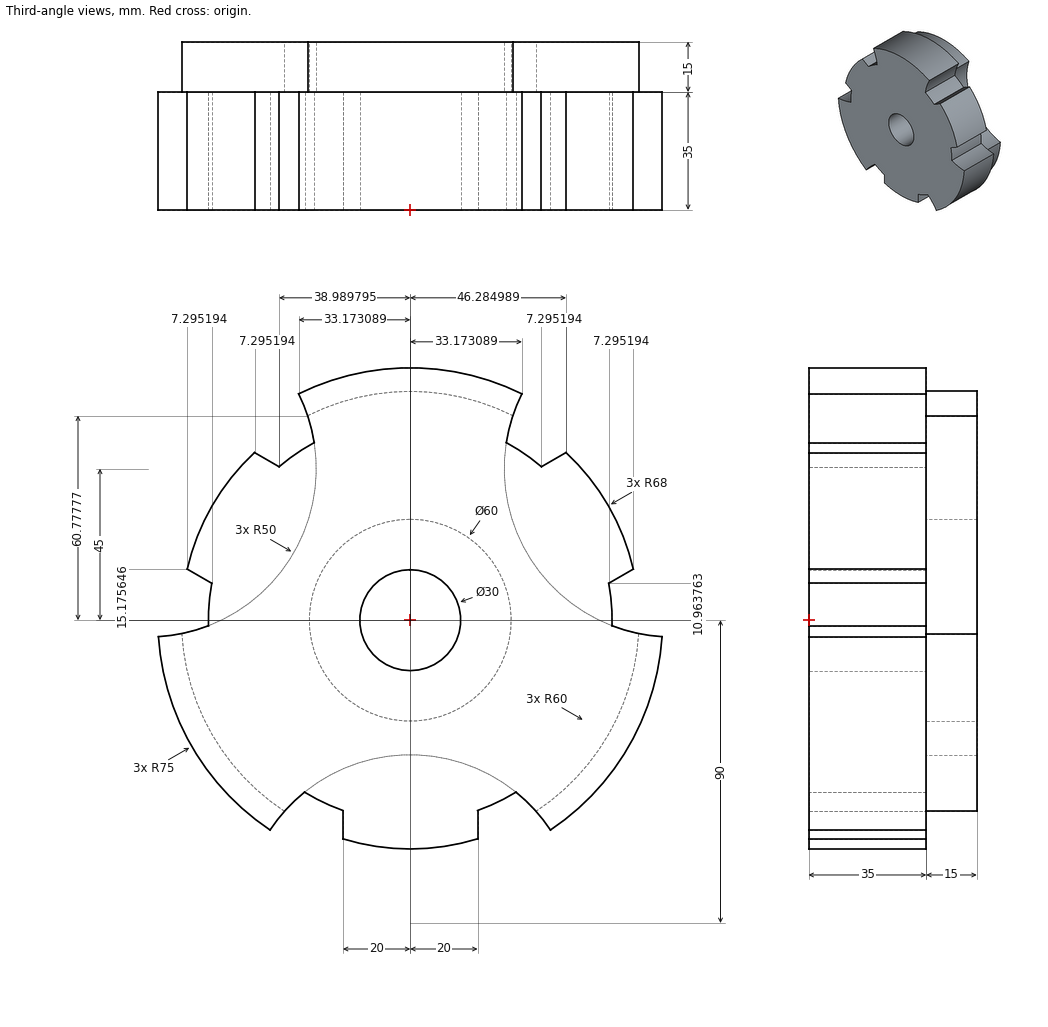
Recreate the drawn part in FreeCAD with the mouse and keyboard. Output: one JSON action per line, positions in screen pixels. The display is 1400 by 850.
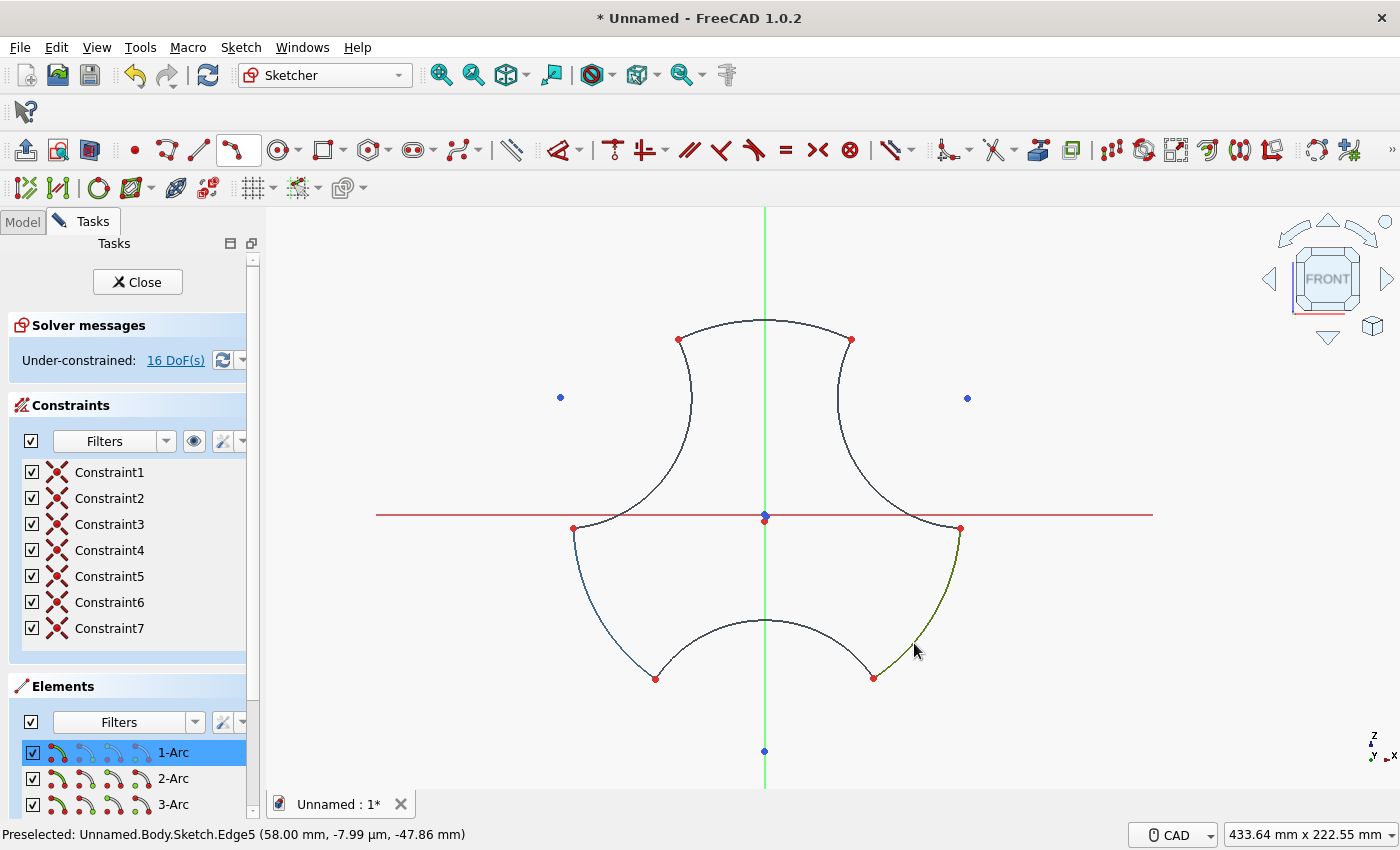
{"action": "key", "text": "c"}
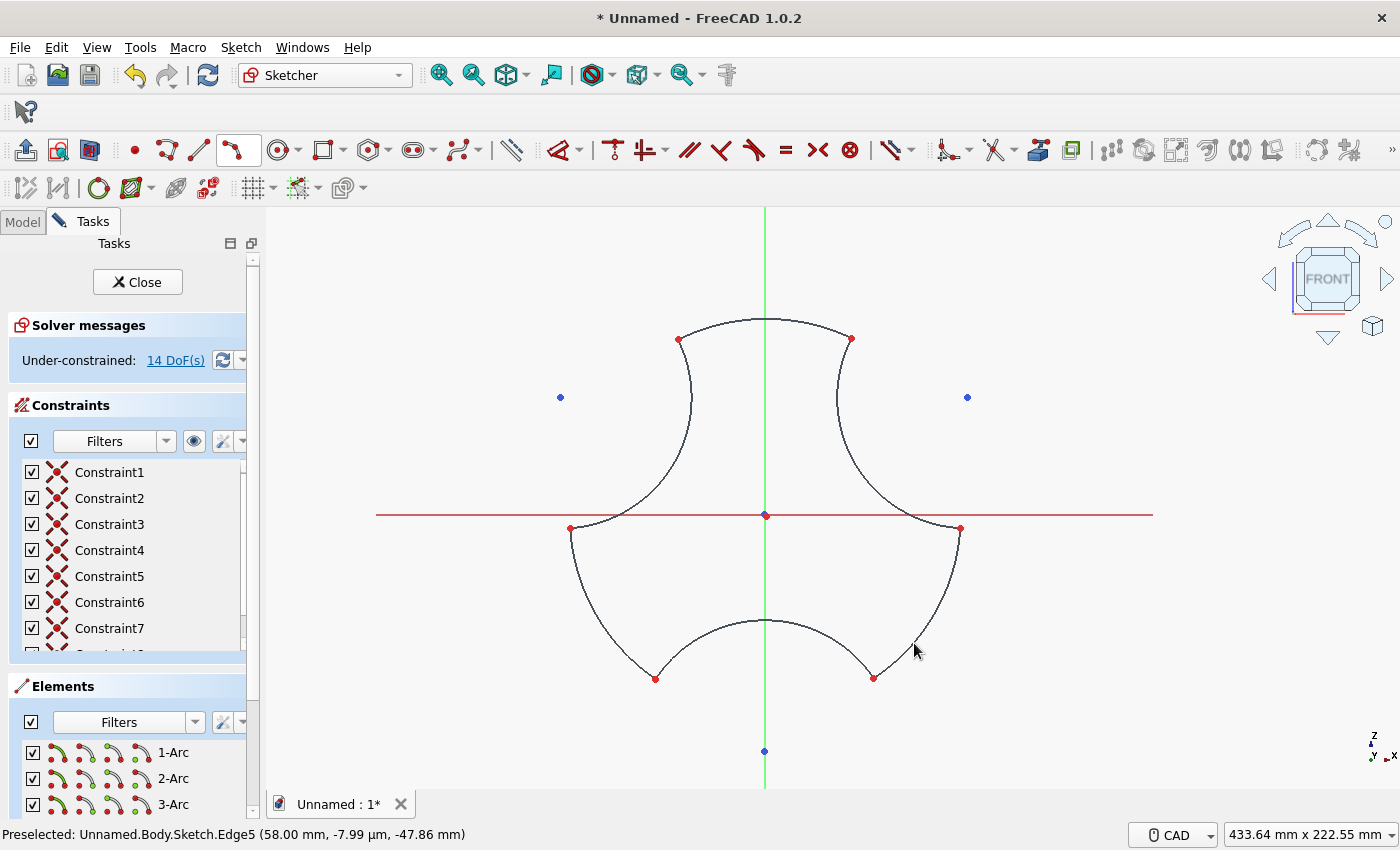
{"action": "left_click_drag", "start_coordinate": [755, 505], "coordinate": [776, 527]}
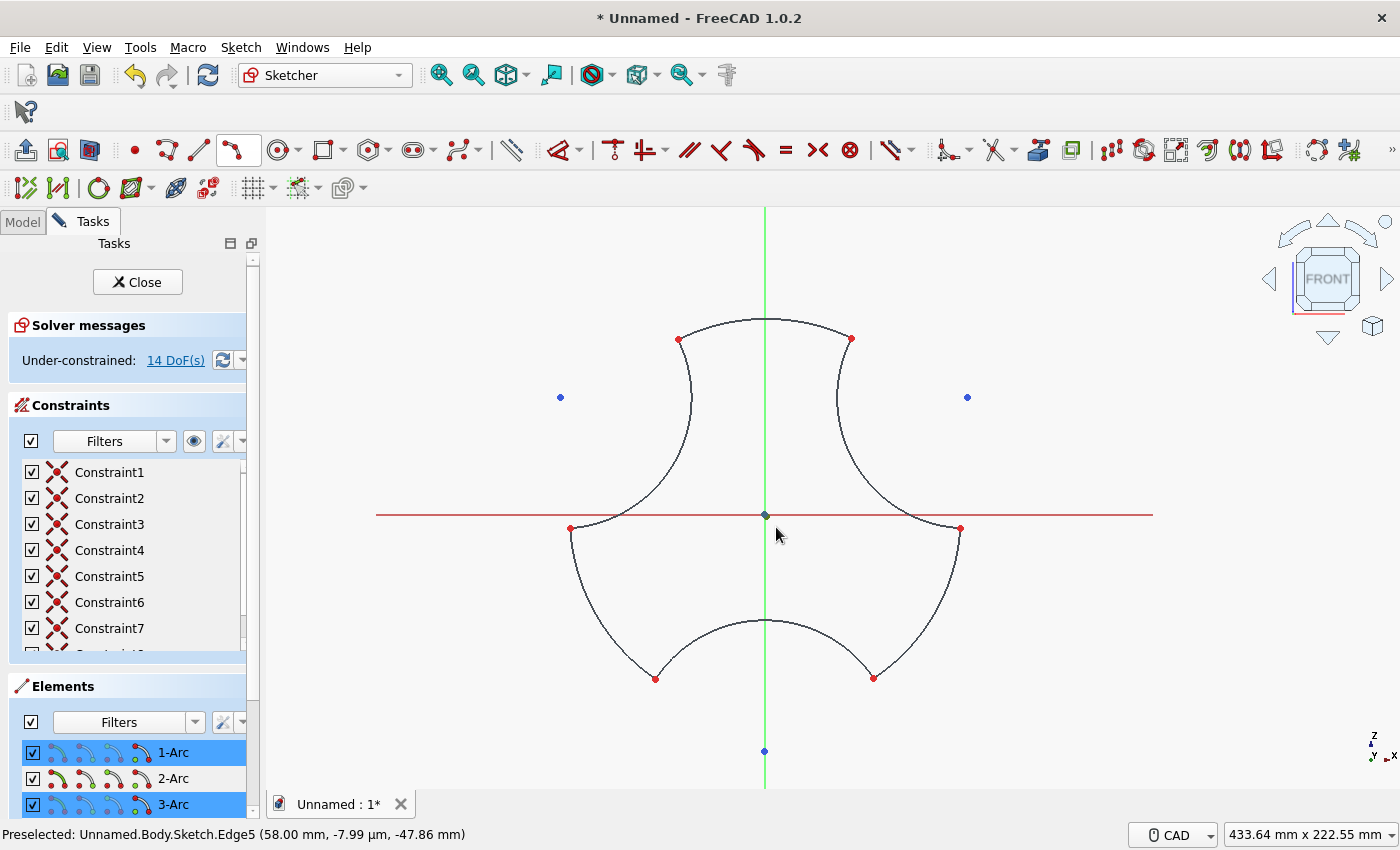
{"action": "left_click", "coordinate": [614, 150]}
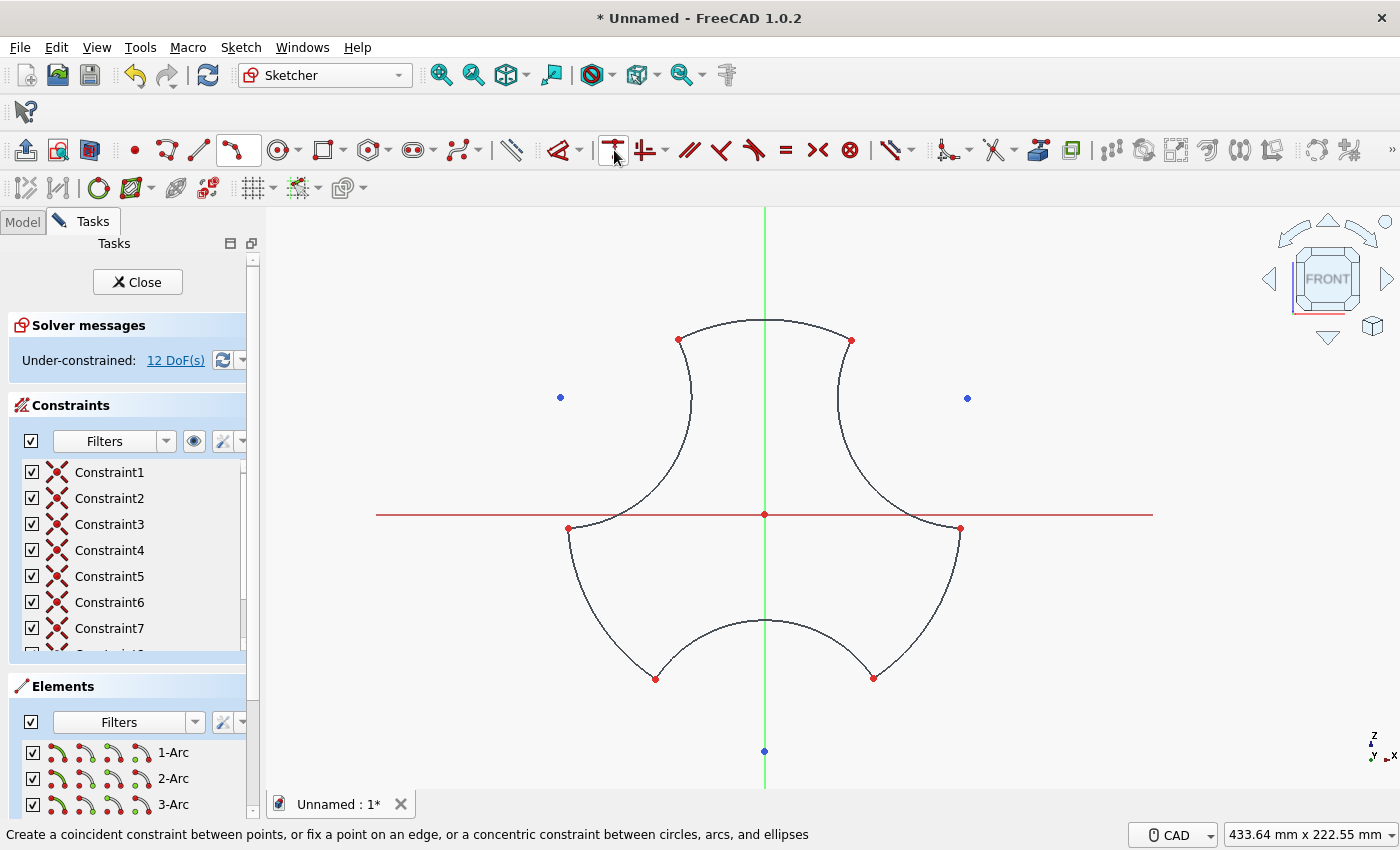
{"action": "left_click", "coordinate": [579, 581]}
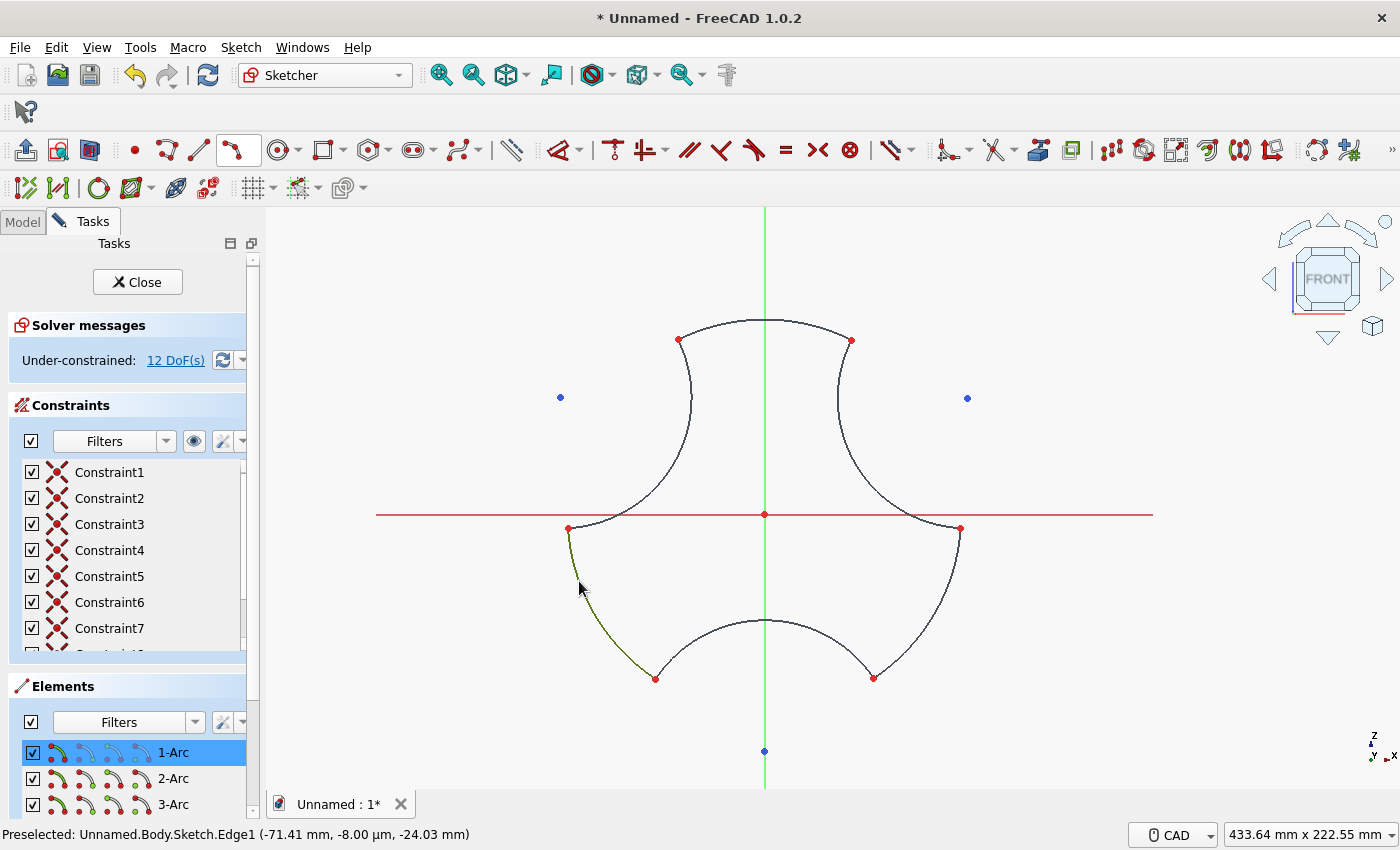
{"action": "left_click", "coordinate": [801, 323]}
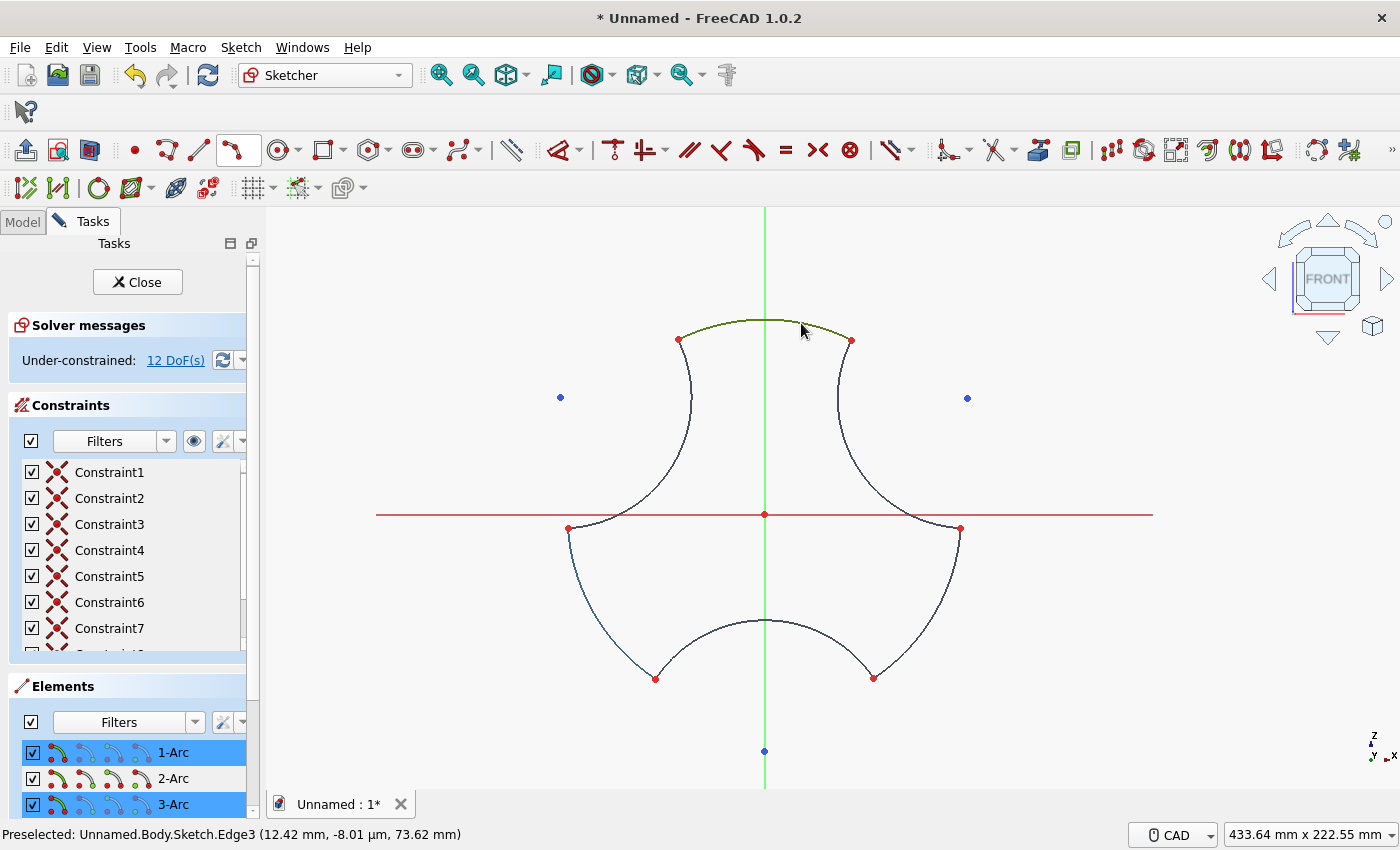
{"action": "left_click", "coordinate": [914, 643]}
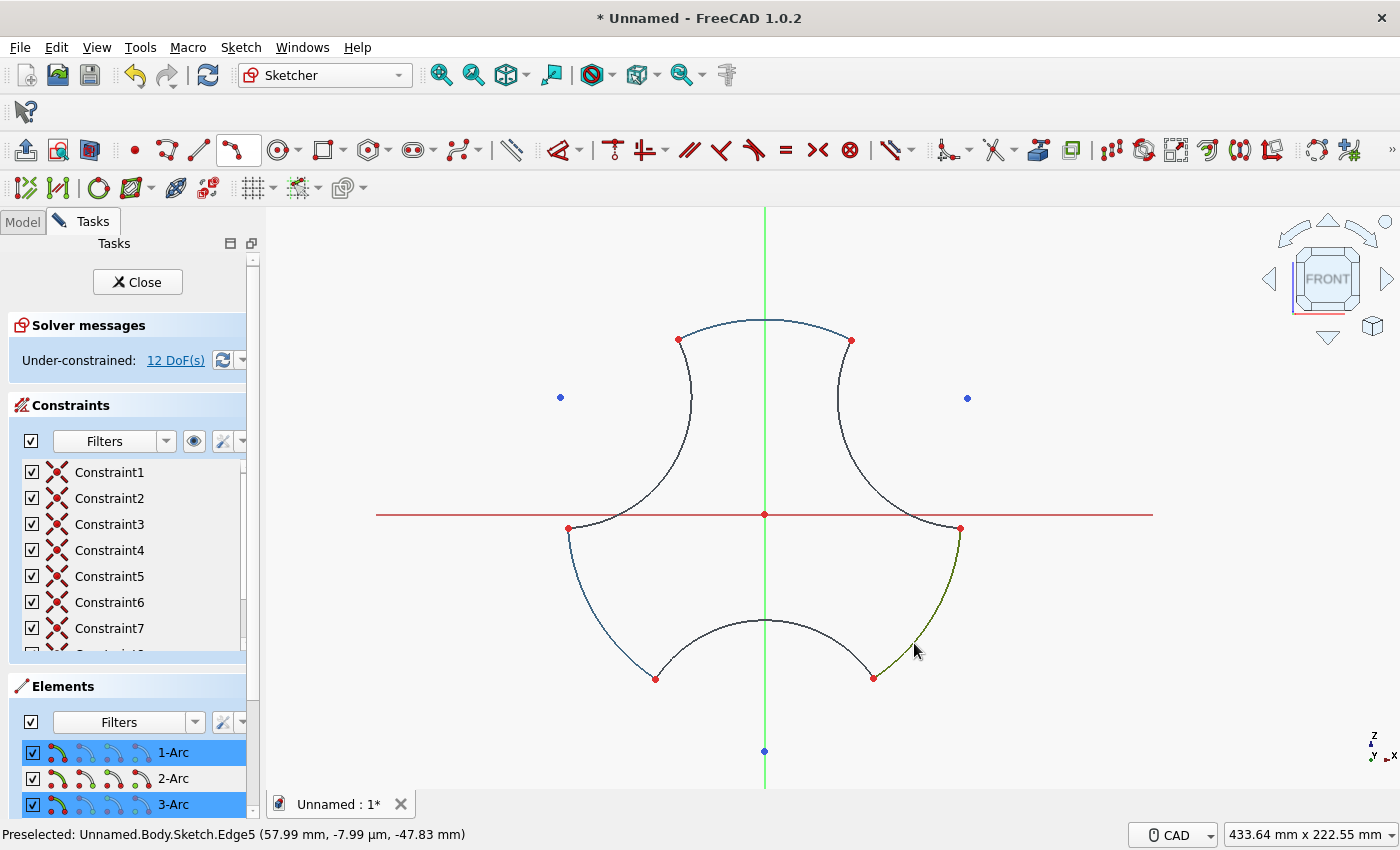
{"action": "left_click", "coordinate": [786, 150]}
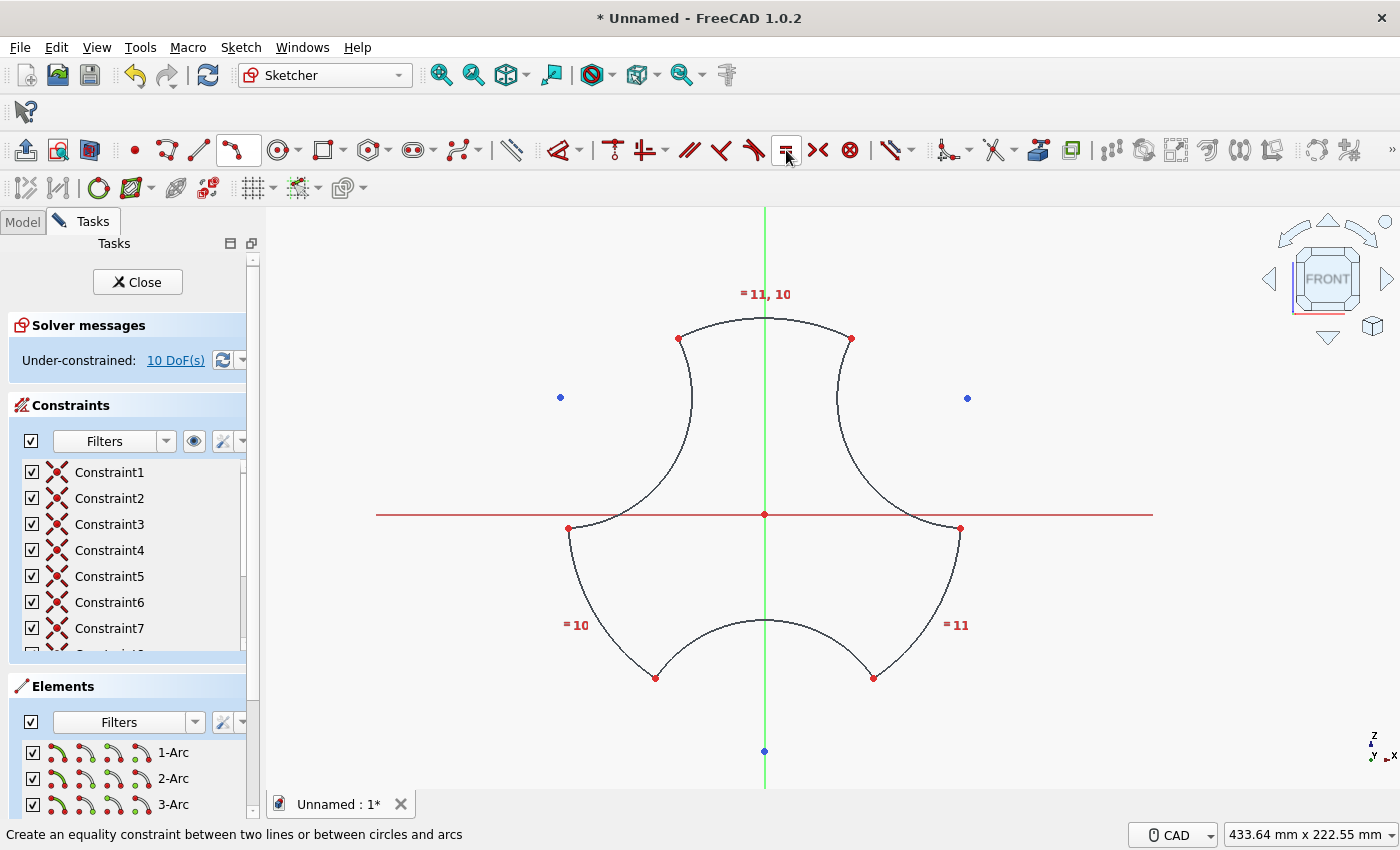
{"action": "left_click", "coordinate": [640, 502]}